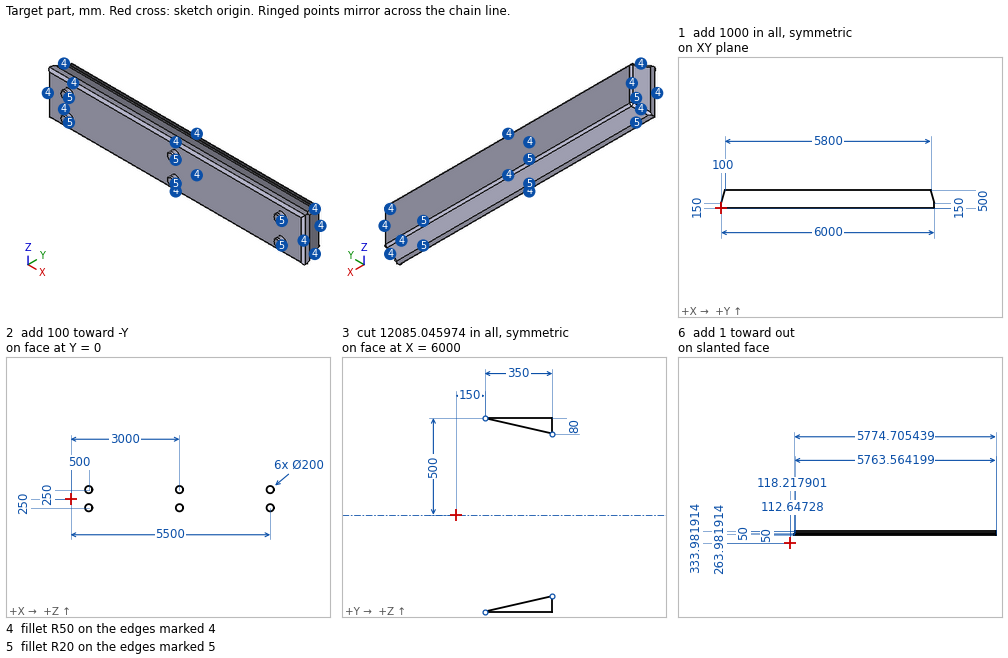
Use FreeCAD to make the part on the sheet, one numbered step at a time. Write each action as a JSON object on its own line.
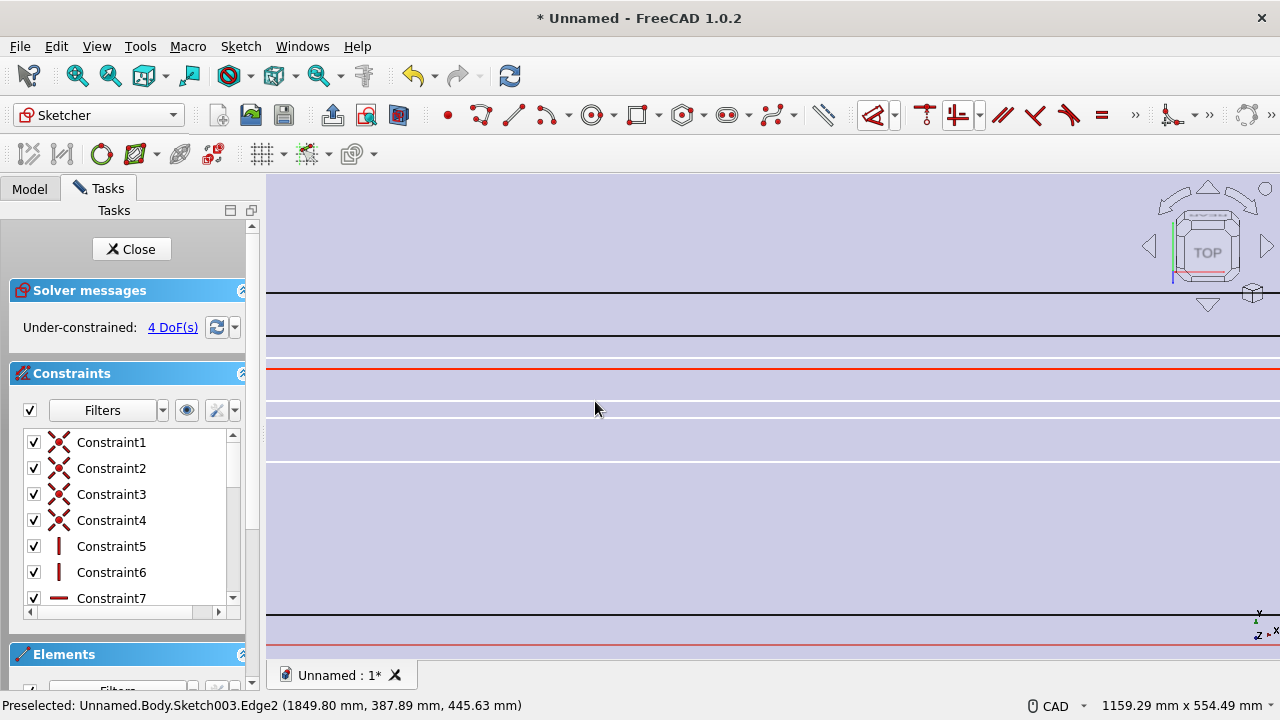
{"action": "scroll", "coordinate": [599, 406], "scroll_direction": "down", "scroll_amount": 11}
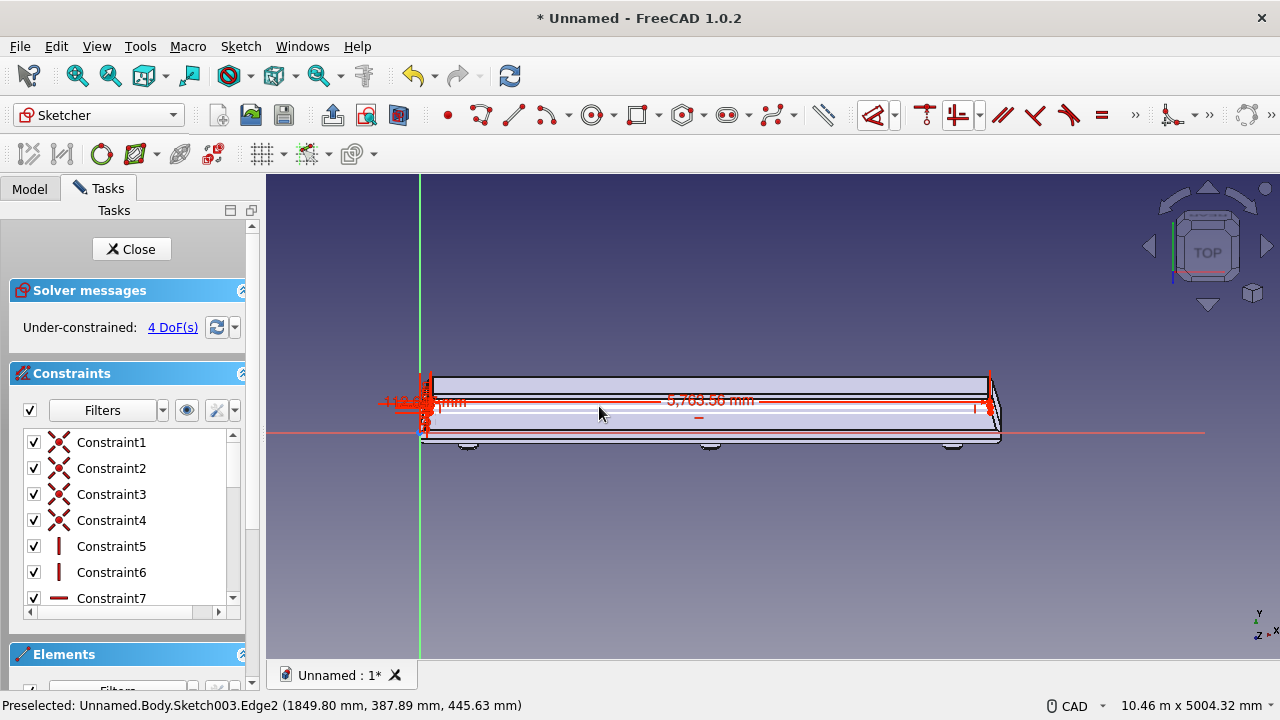
{"action": "scroll", "coordinate": [598, 413], "scroll_direction": "up", "scroll_amount": 6}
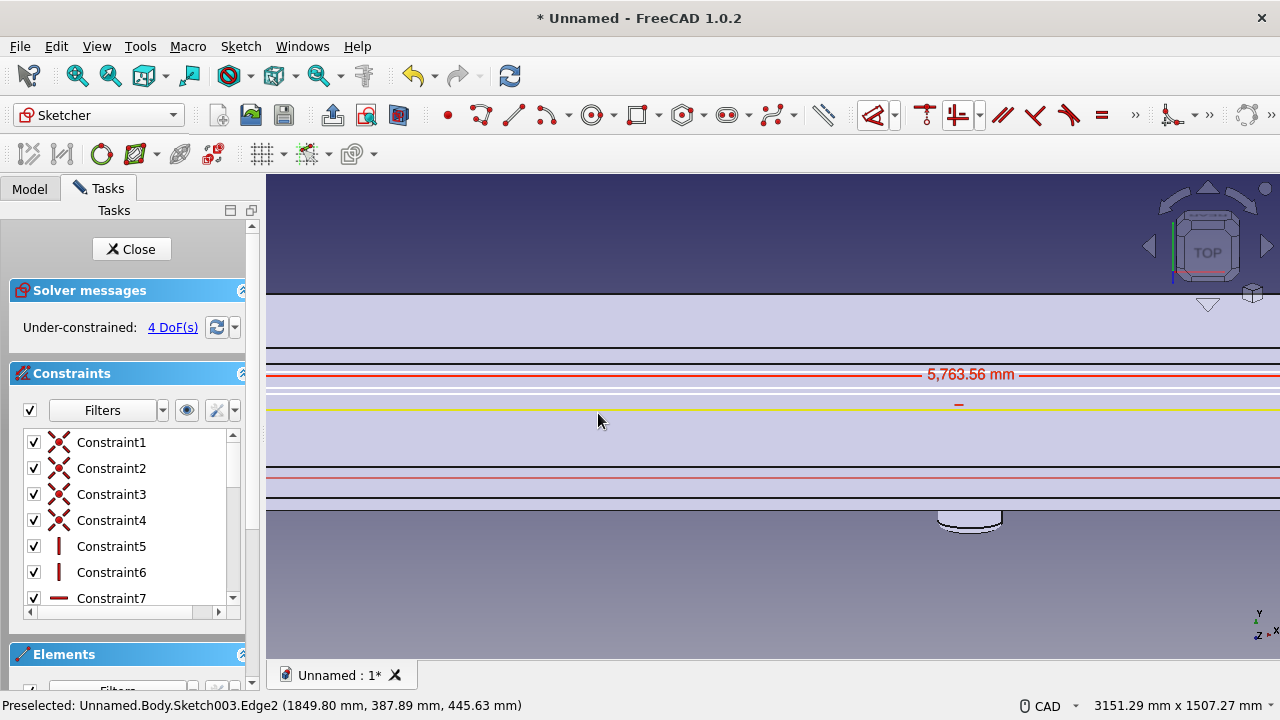
{"action": "left_click", "coordinate": [598, 410]}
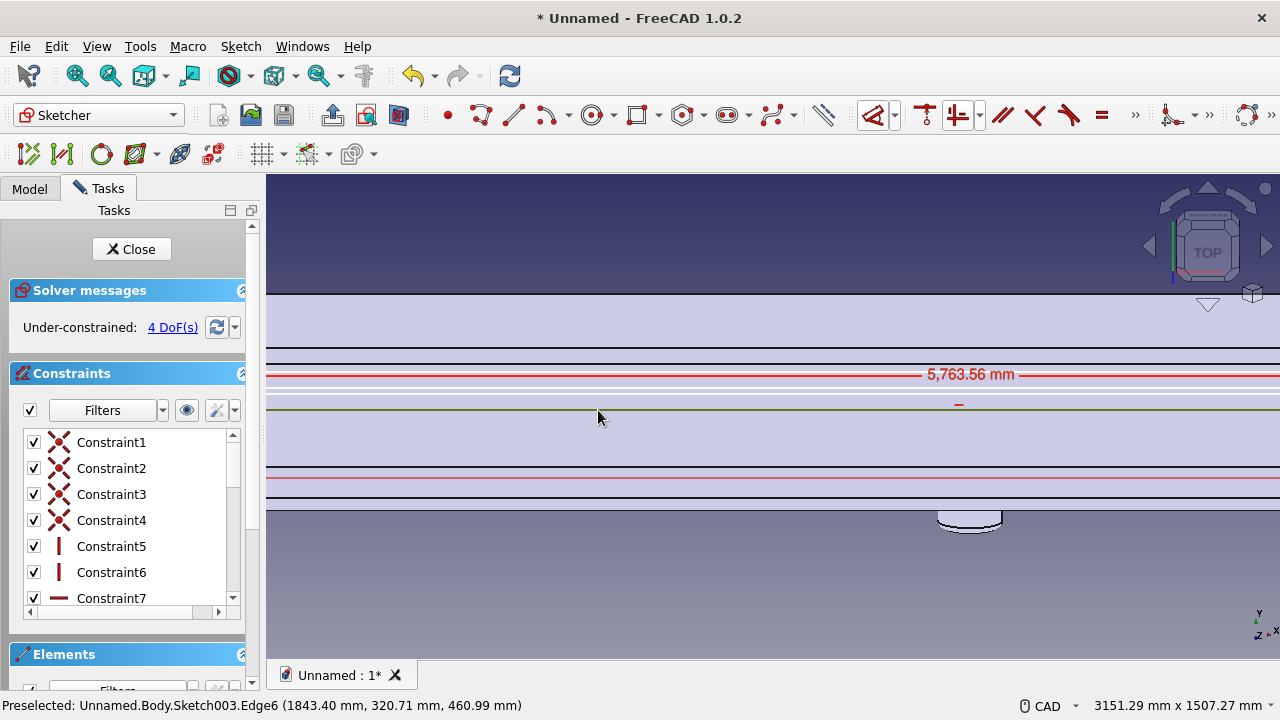
{"action": "left_click", "coordinate": [894, 116]}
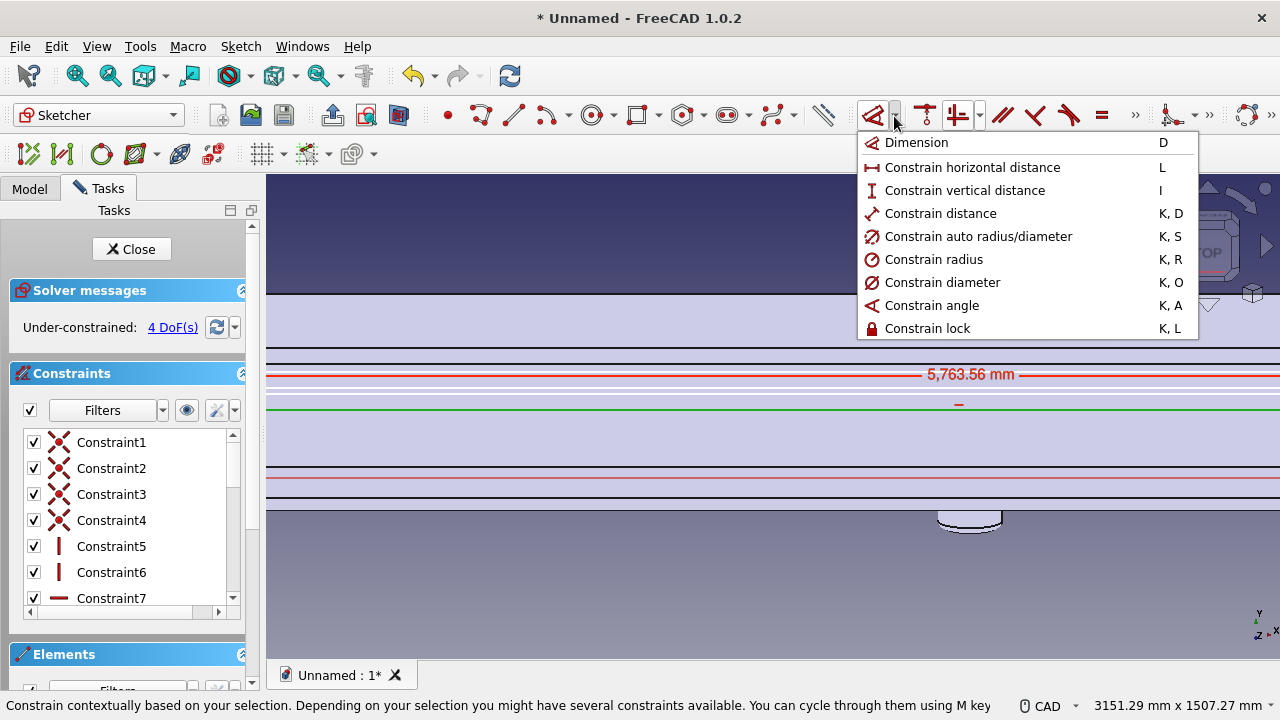
{"action": "left_click", "coordinate": [1028, 168]}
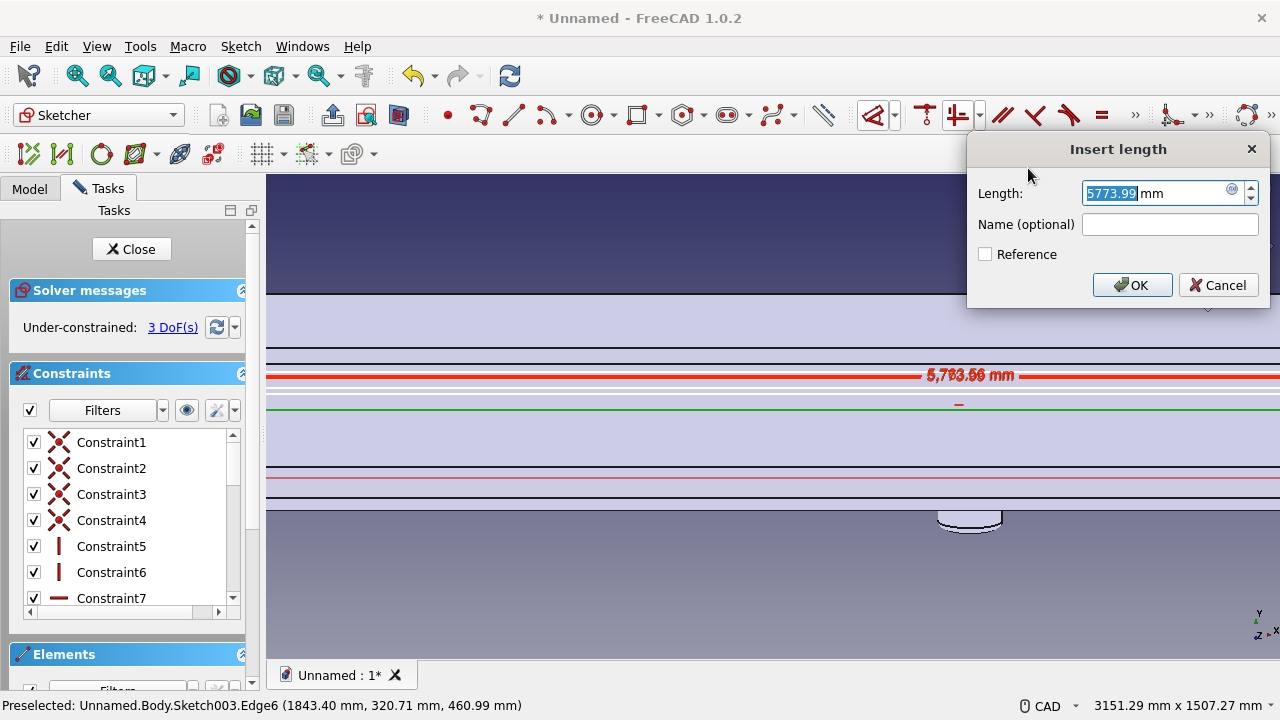
{"action": "type", "text": "5774.705439"}
{"action": "key", "text": "Return"}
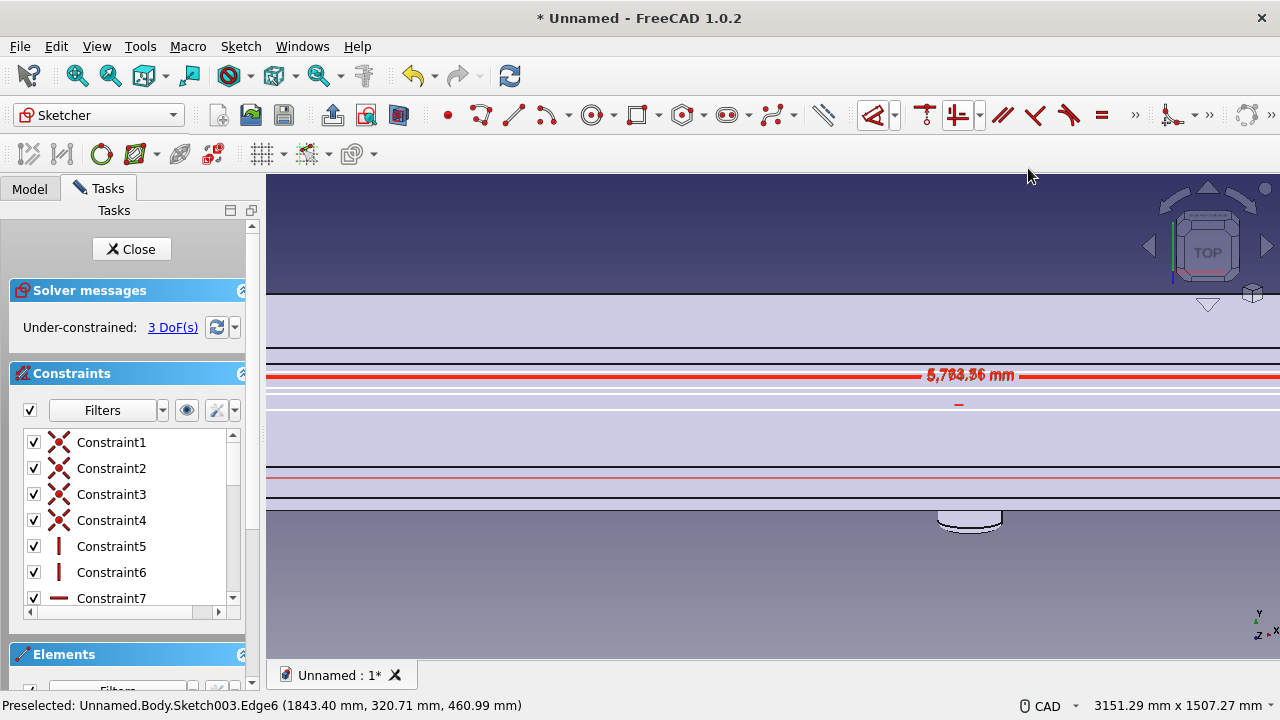
{"action": "scroll", "coordinate": [598, 413], "scroll_direction": "down", "scroll_amount": 6}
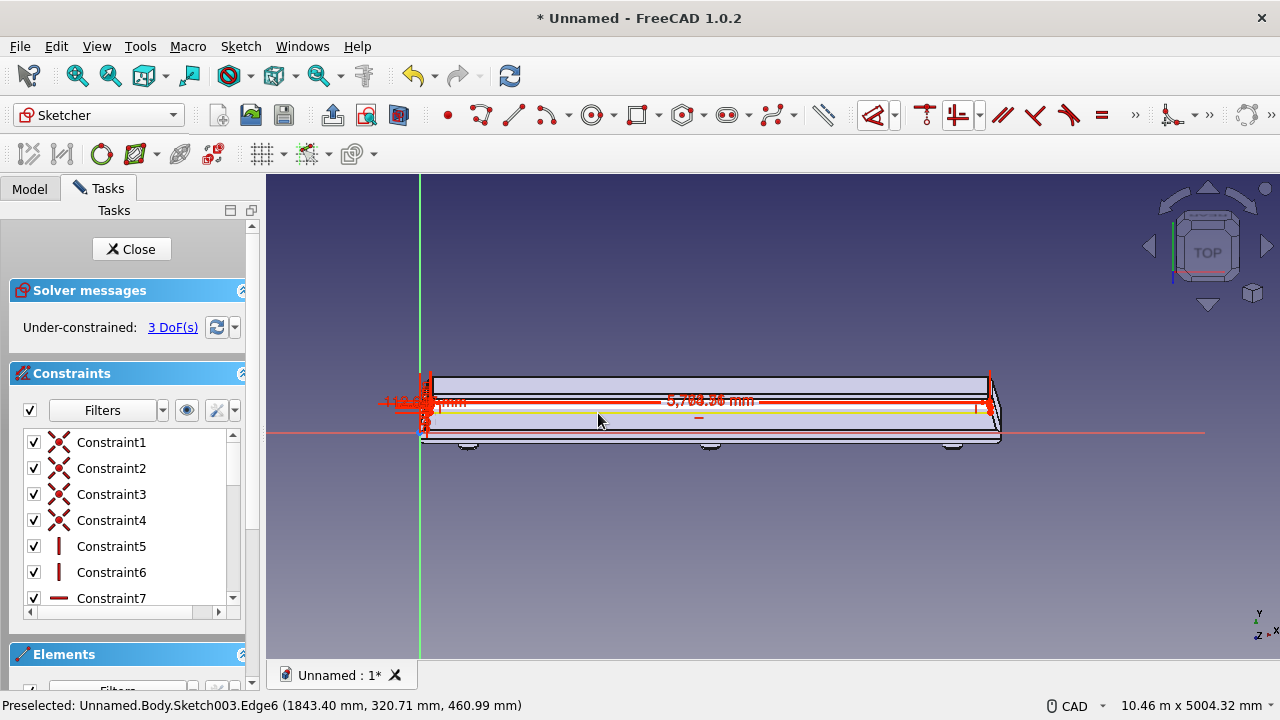
{"action": "scroll", "coordinate": [431, 401], "scroll_direction": "up", "scroll_amount": 7}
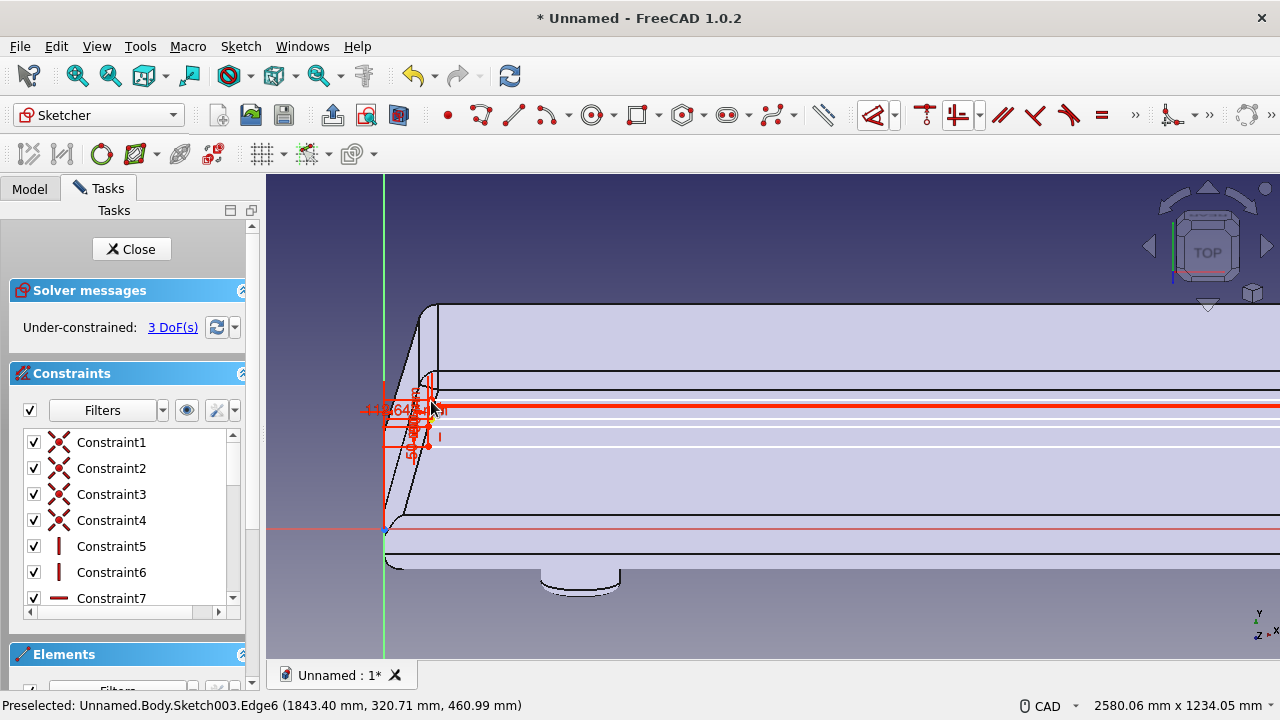
{"action": "left_click", "coordinate": [432, 400]}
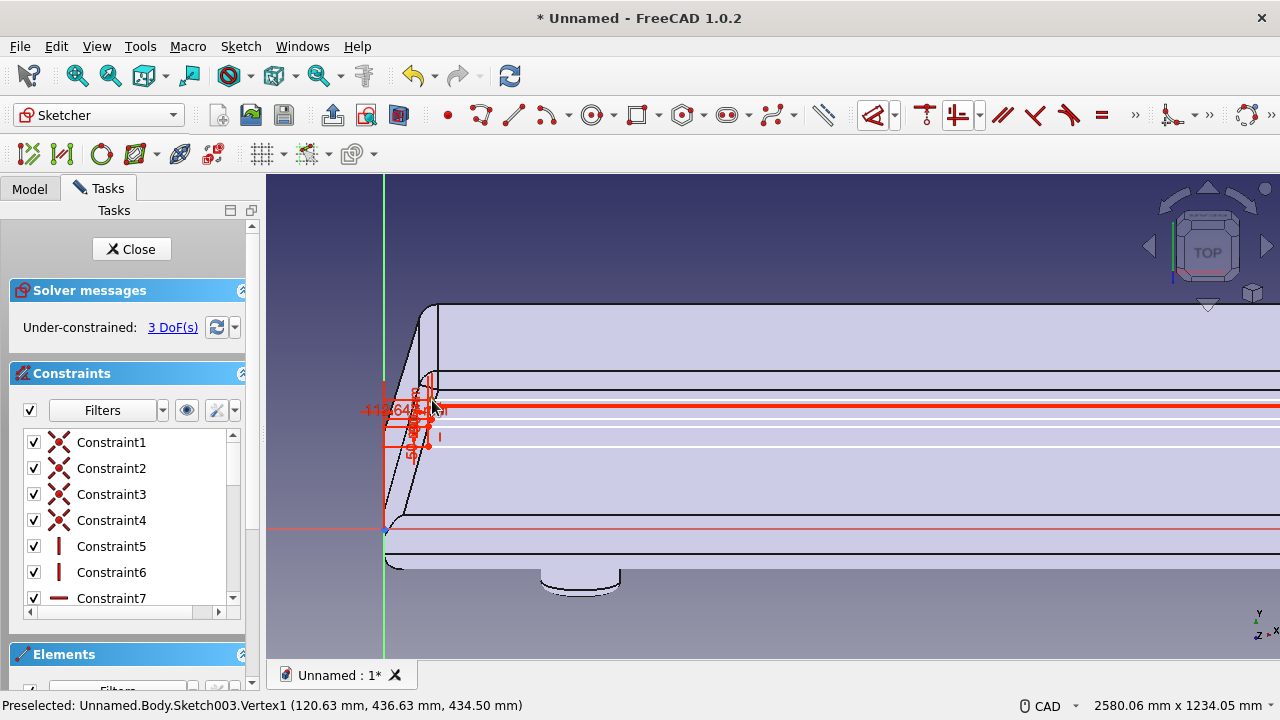
{"action": "key", "text": "l"}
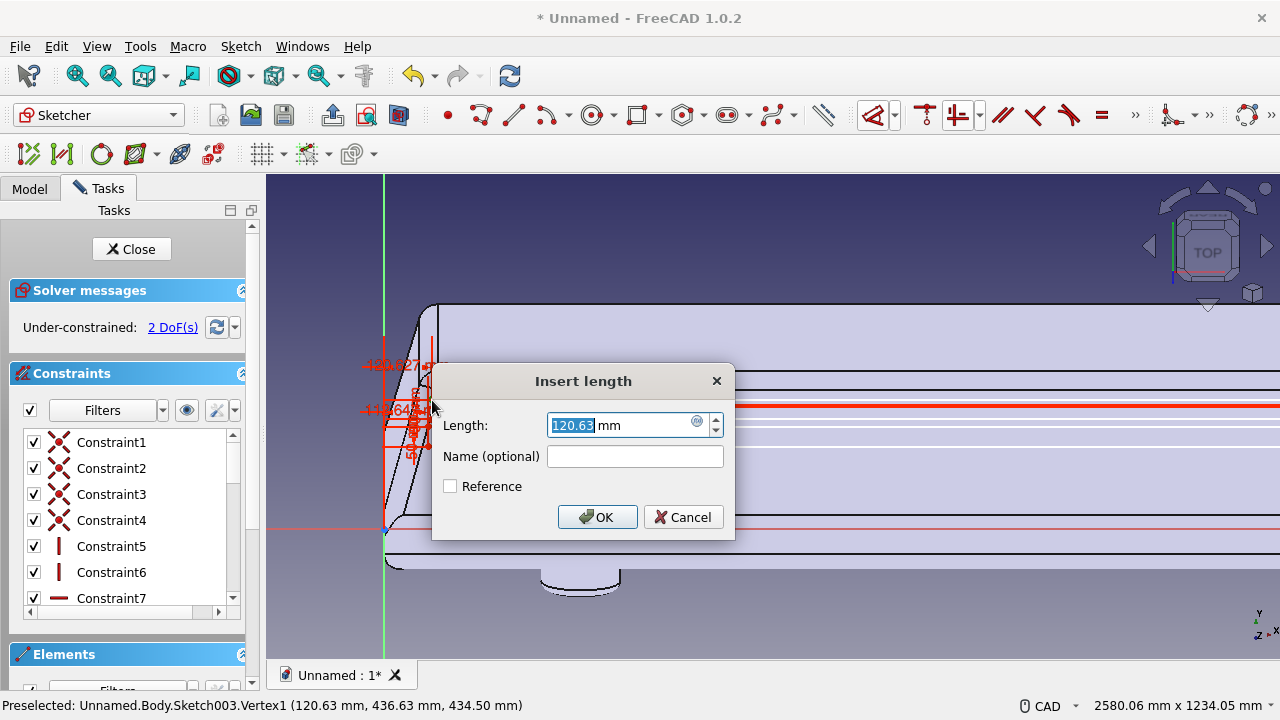
{"action": "type", "text": "118.217901"}
{"action": "key", "text": "Return"}